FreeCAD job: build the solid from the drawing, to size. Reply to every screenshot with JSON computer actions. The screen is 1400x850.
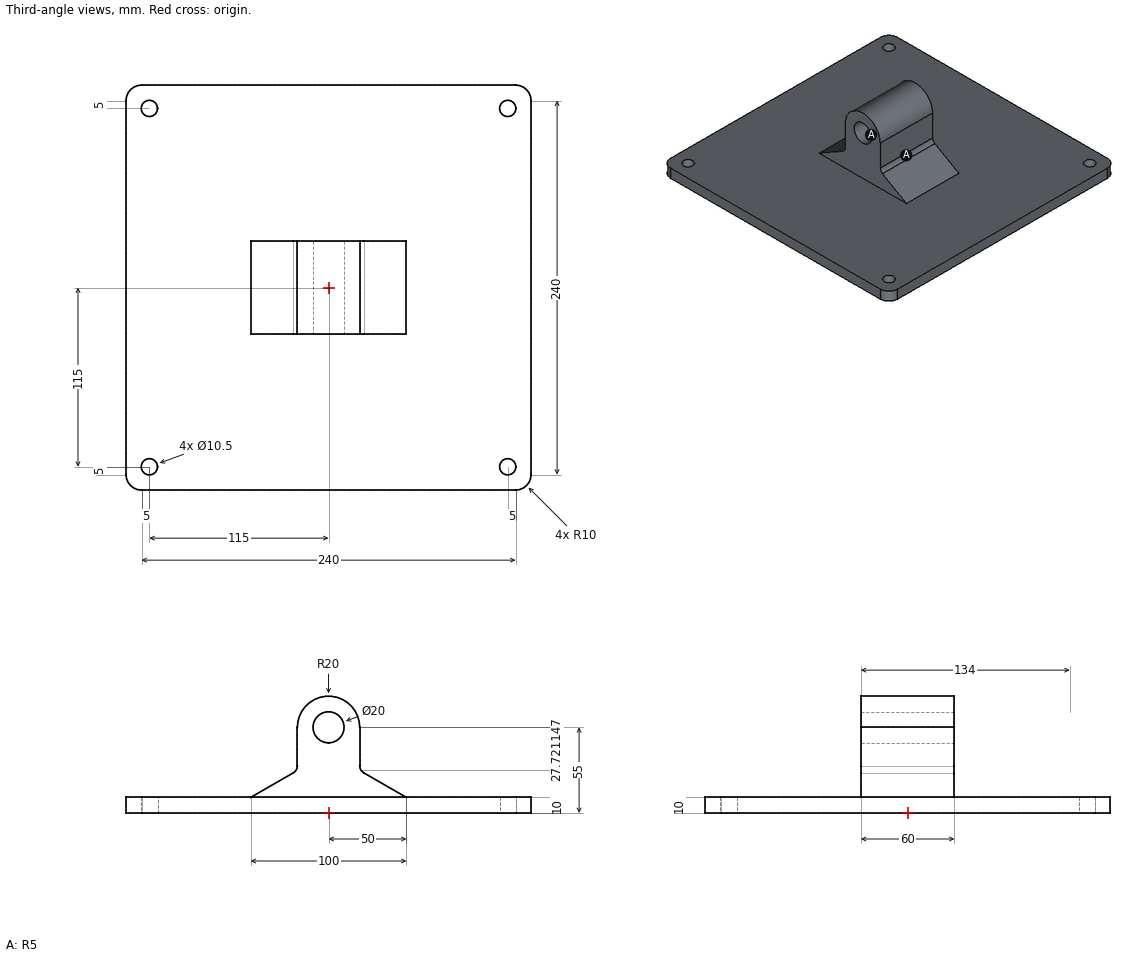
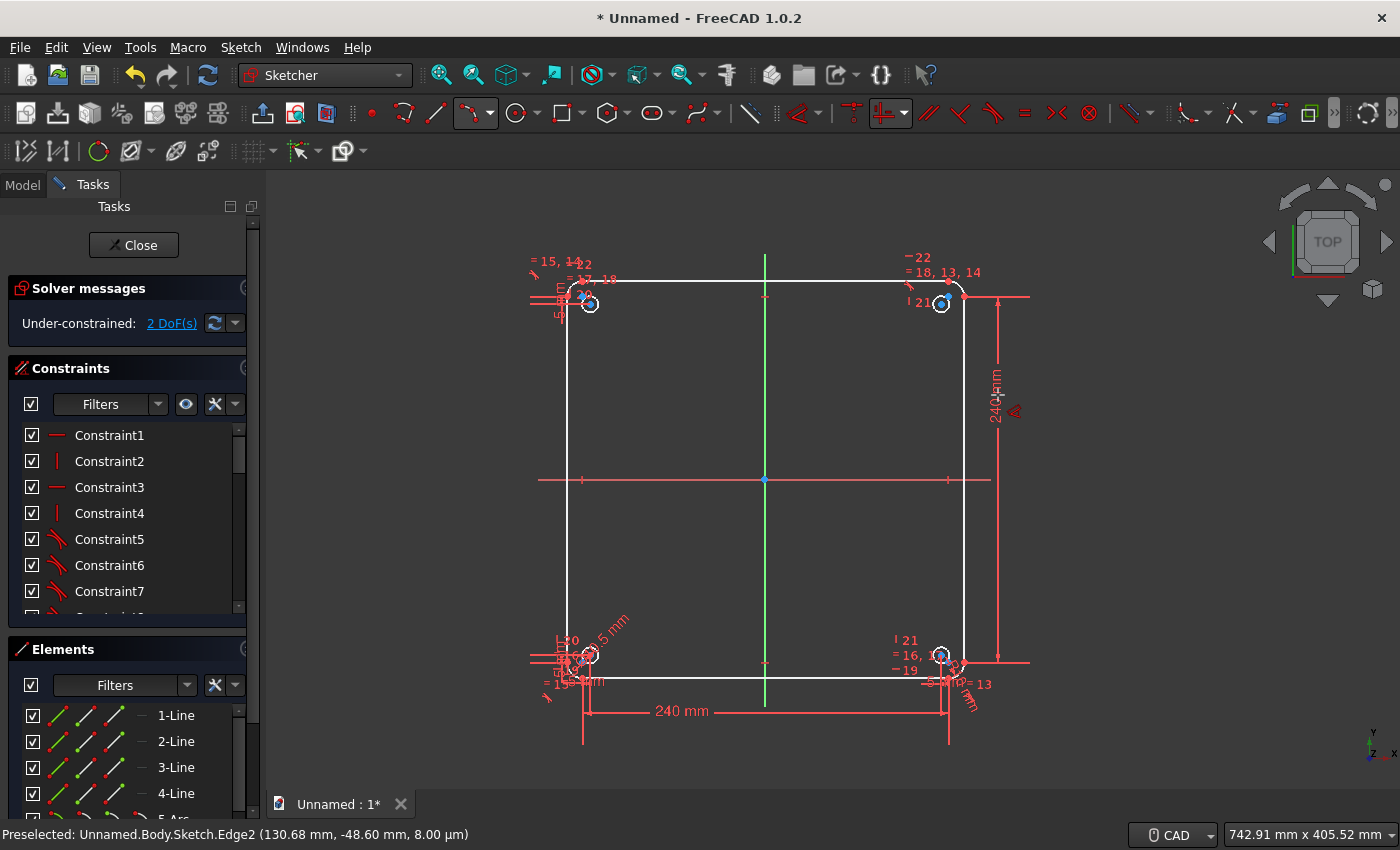
{"action": "left_click", "coordinate": [590, 655]}
{"action": "left_click", "coordinate": [677, 446]}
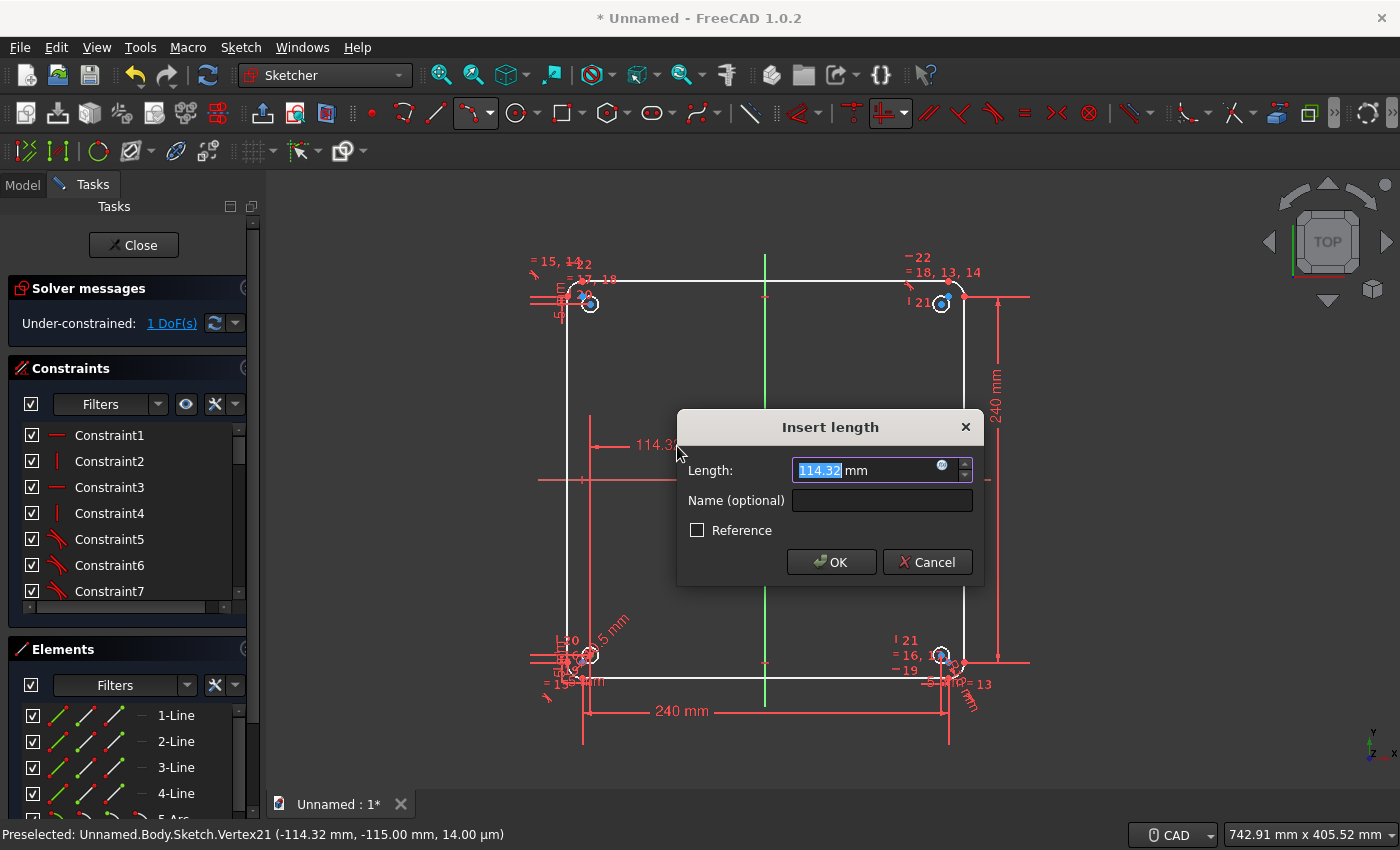
{"action": "type", "text": "115"}
{"action": "key", "text": "Return"}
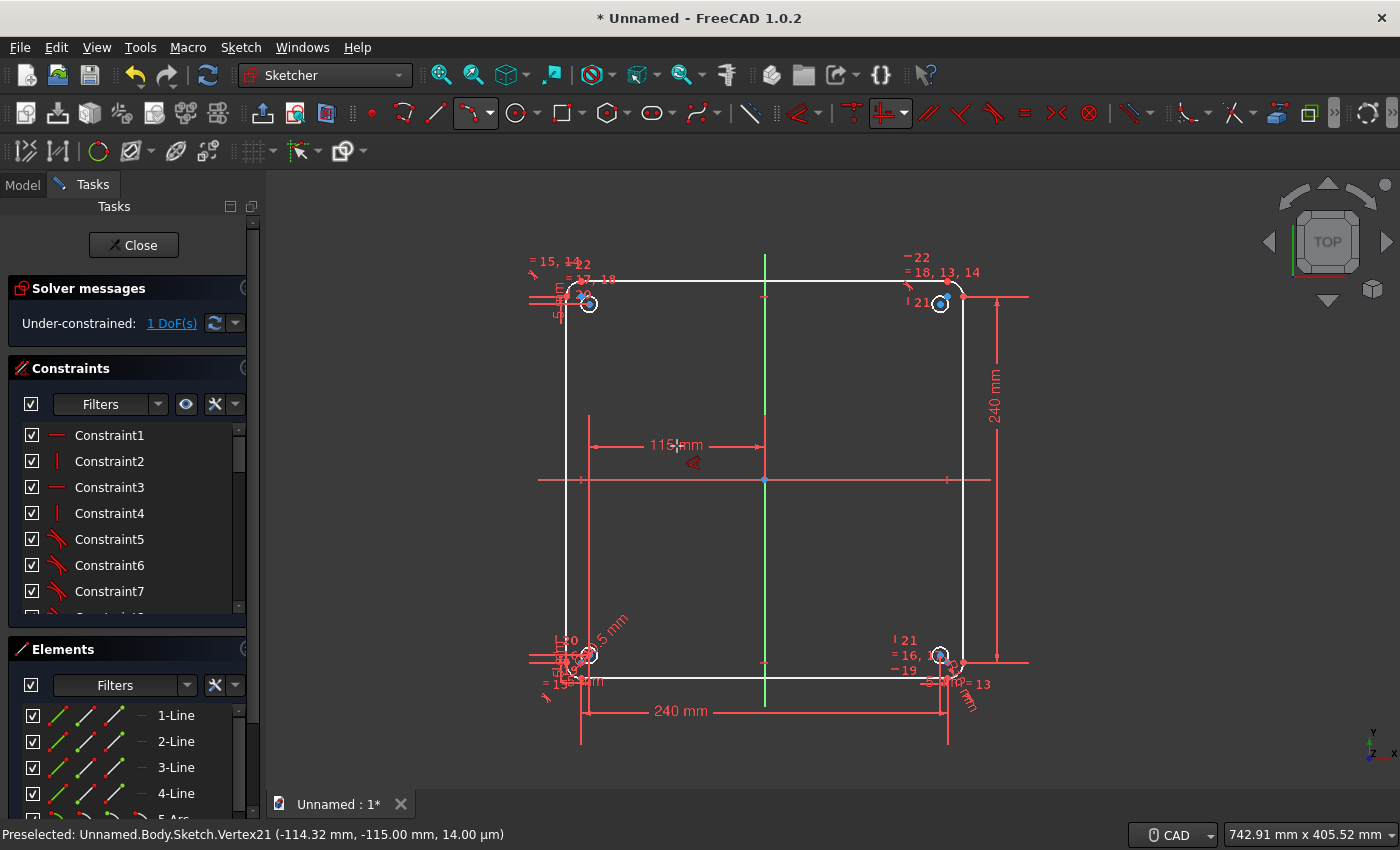
{"action": "left_click", "coordinate": [589, 655]}
{"action": "left_click", "coordinate": [799, 568]}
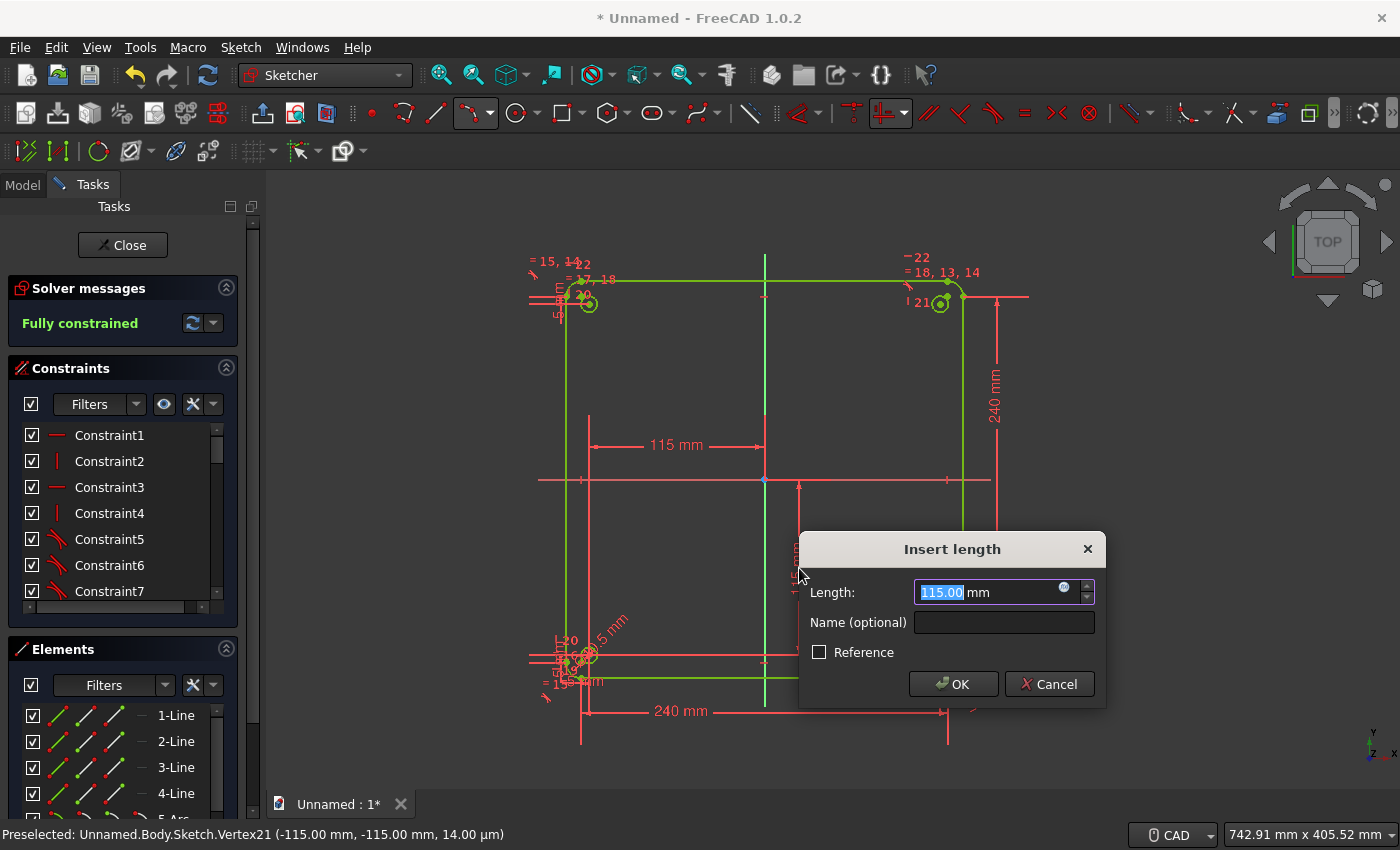
{"action": "type", "text": "115"}
{"action": "key", "text": "Return"}
{"action": "key", "text": "Escape"}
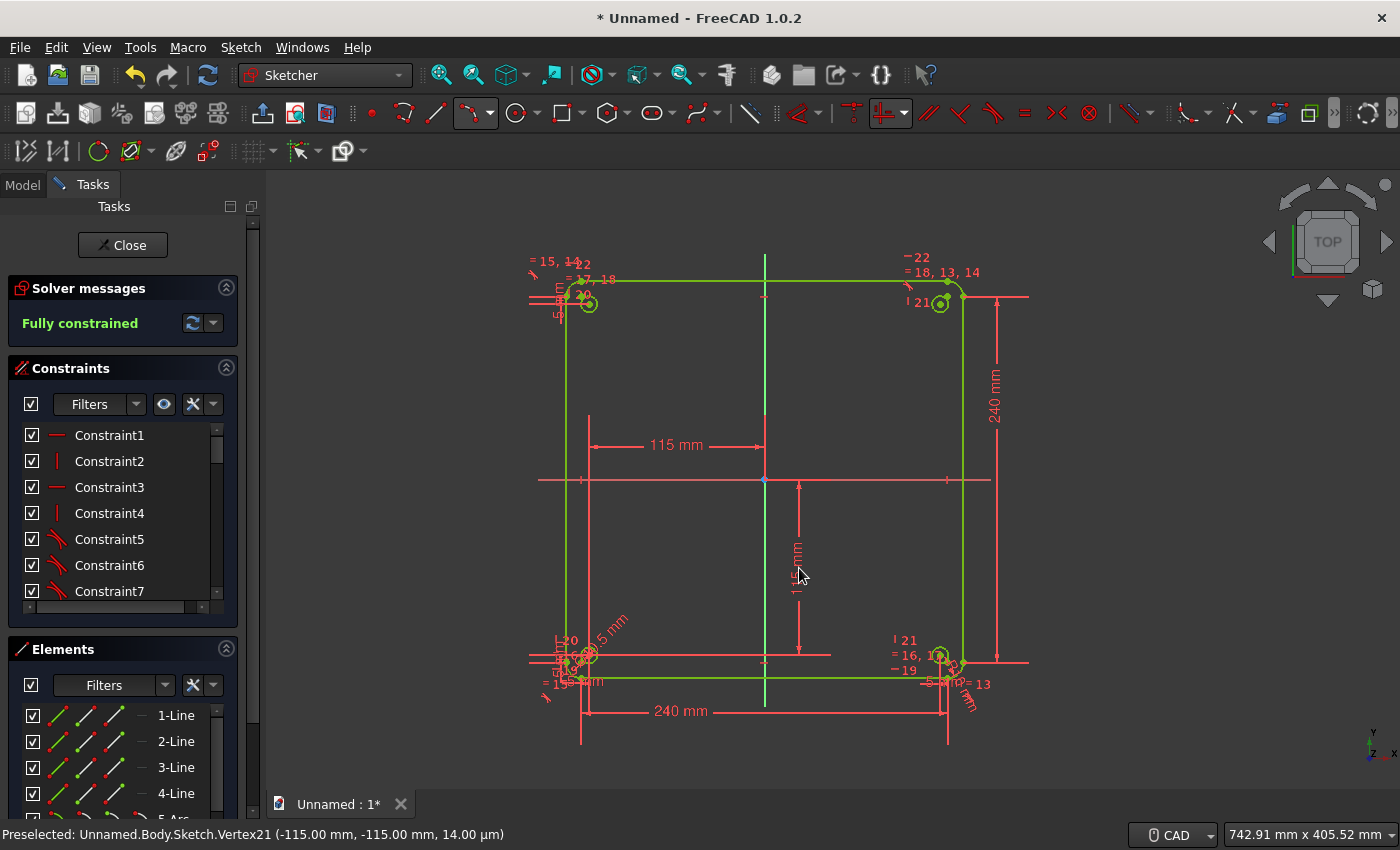
{"action": "left_click", "coordinate": [123, 245]}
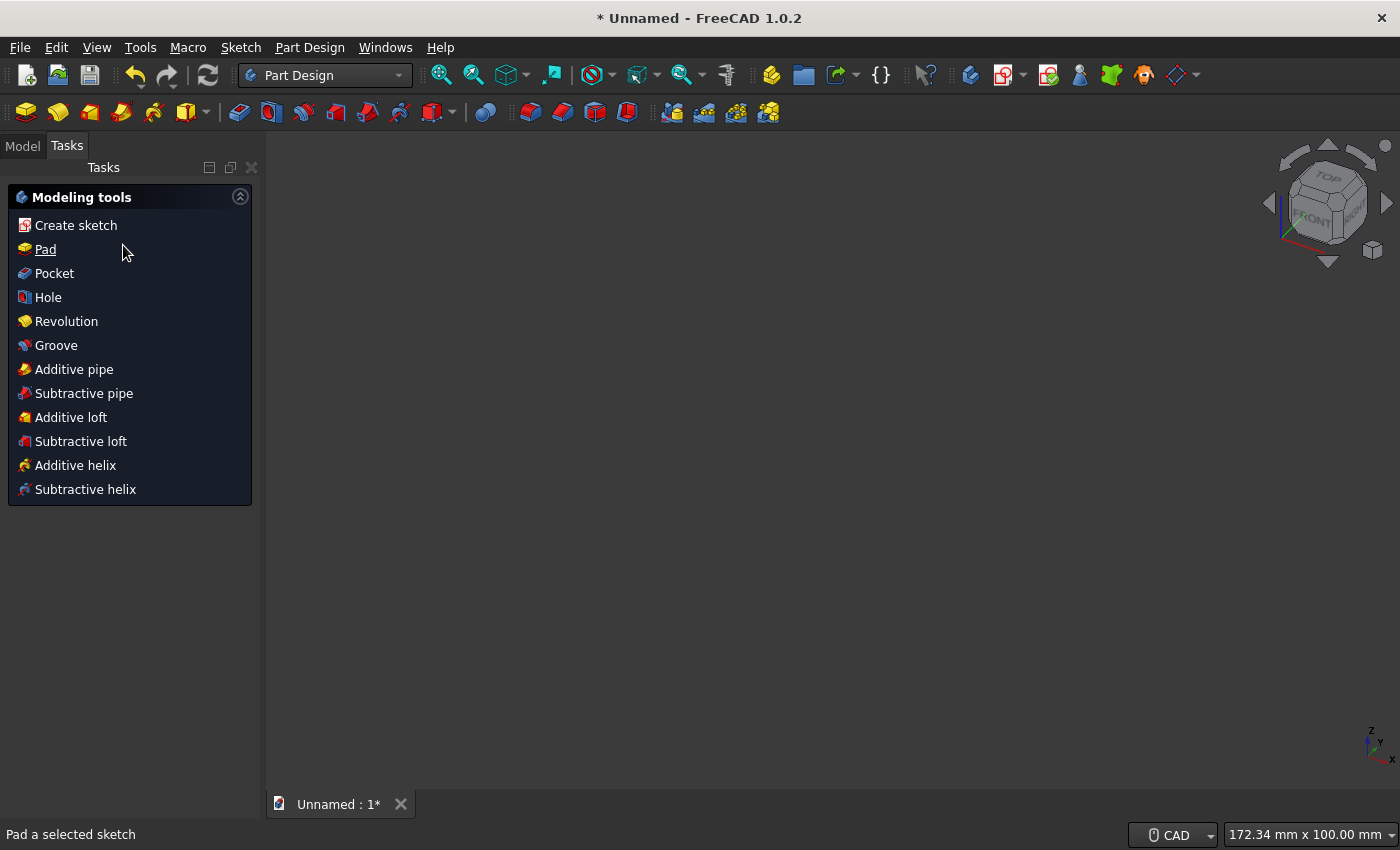
{"action": "left_click", "coordinate": [26, 112]}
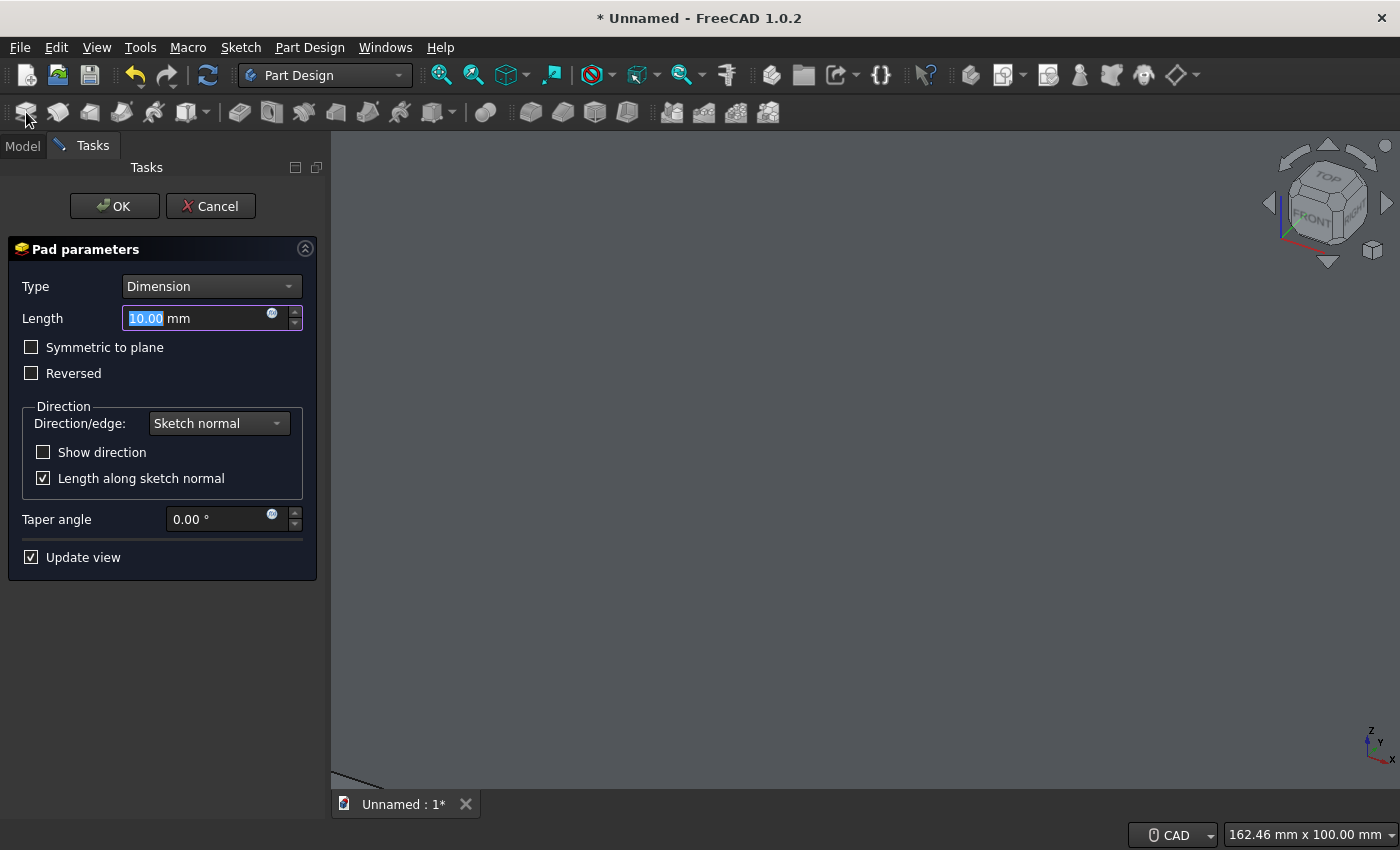
{"action": "type", "text": "10"}
{"action": "key", "text": "Tab"}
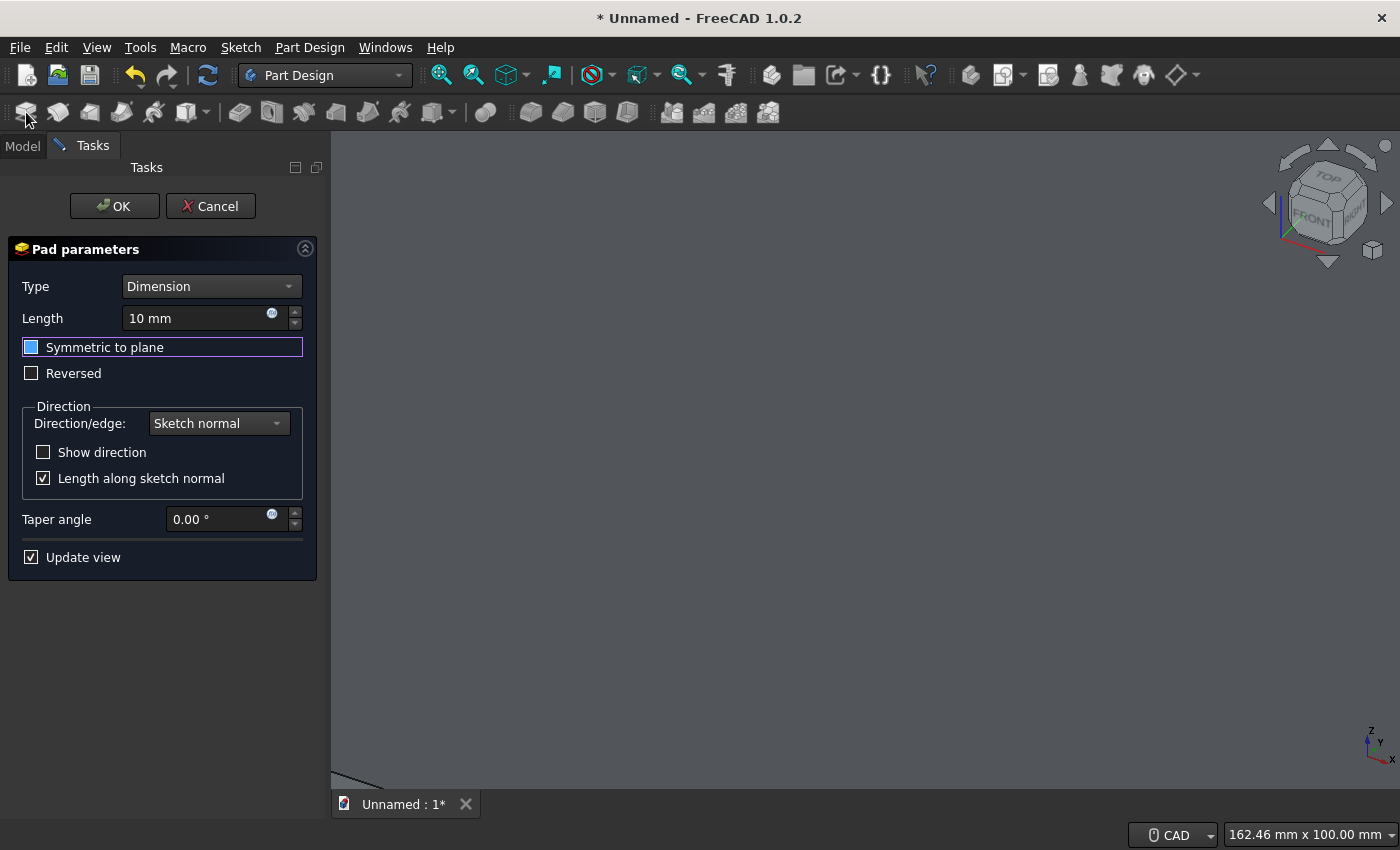
{"action": "left_click", "coordinate": [115, 206]}